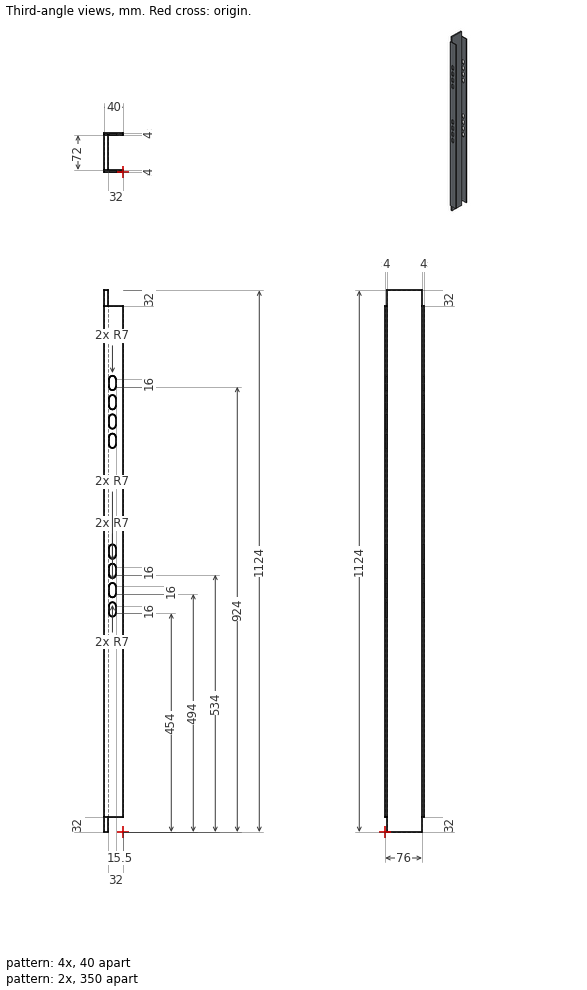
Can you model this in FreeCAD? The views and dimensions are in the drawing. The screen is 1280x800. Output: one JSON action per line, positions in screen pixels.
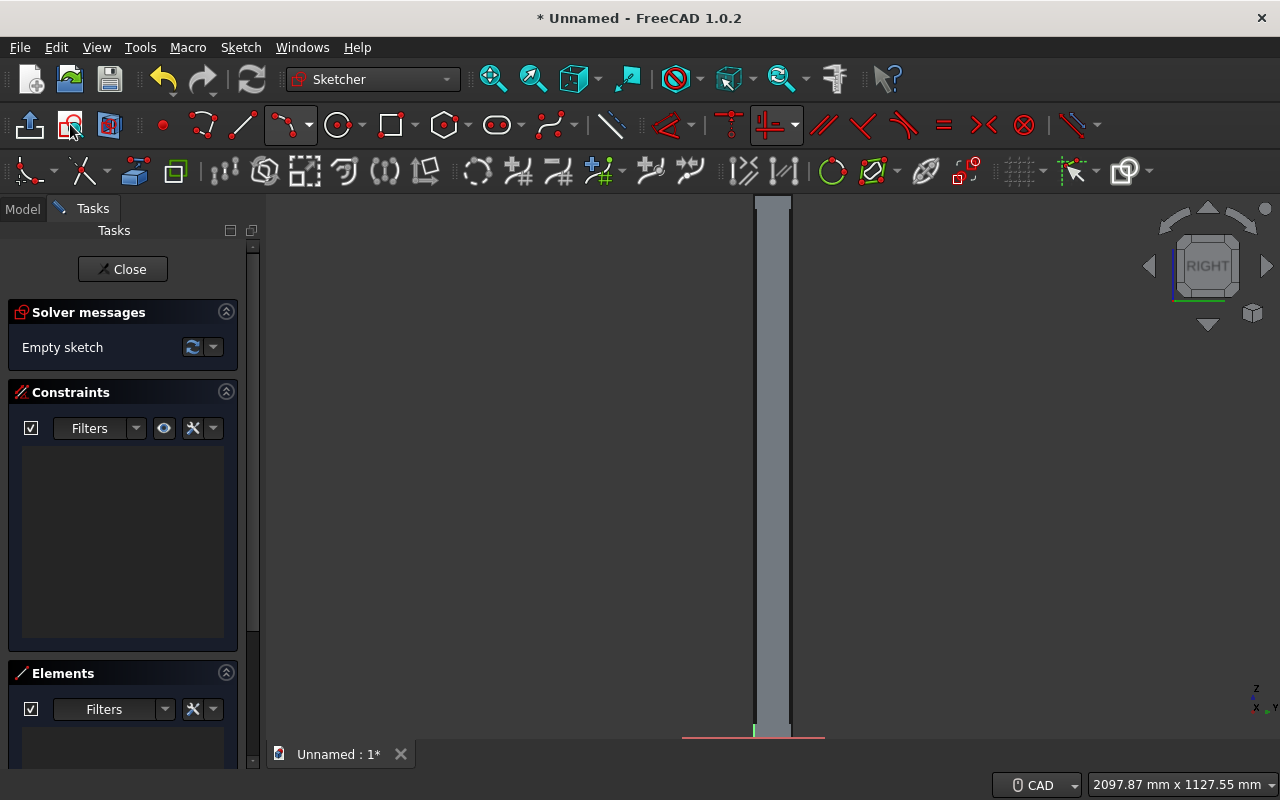
{"action": "scroll", "coordinate": [565, 466], "scroll_direction": "down", "scroll_amount": 2}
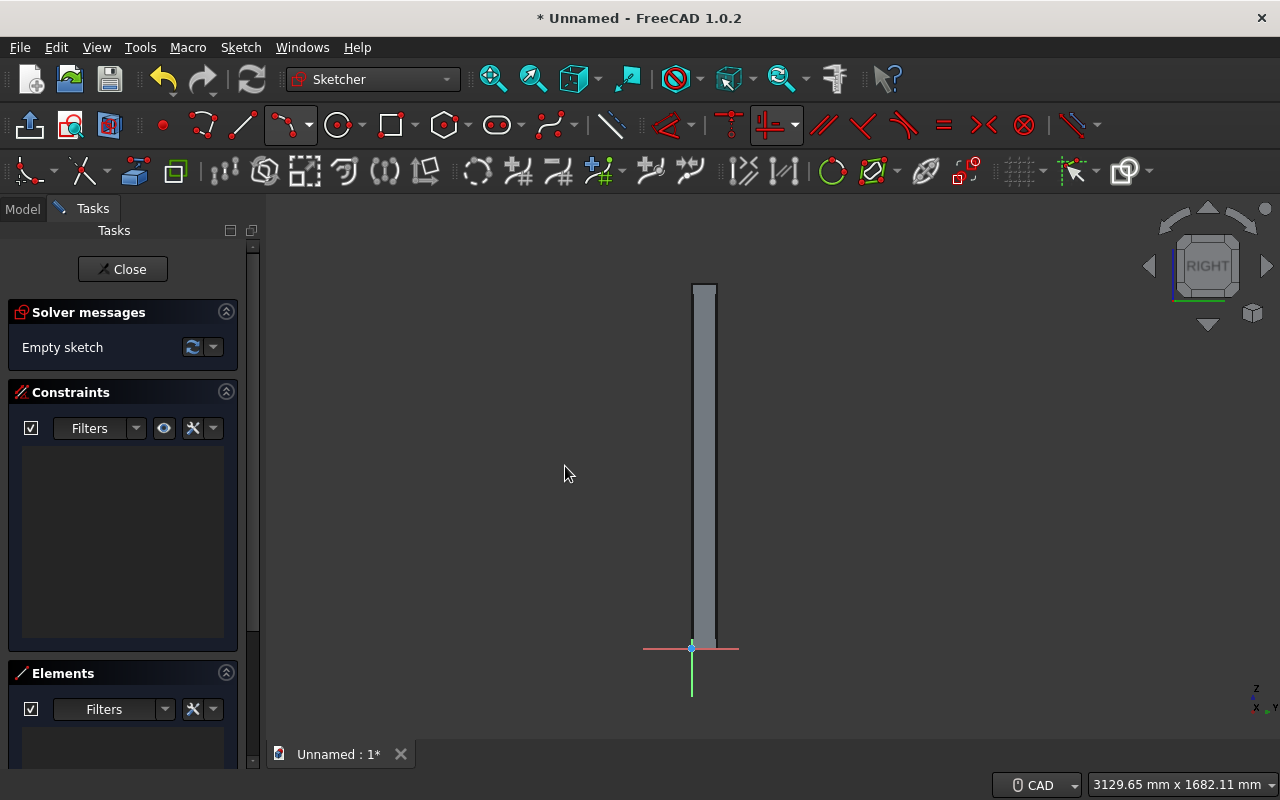
{"action": "key", "text": "g r"}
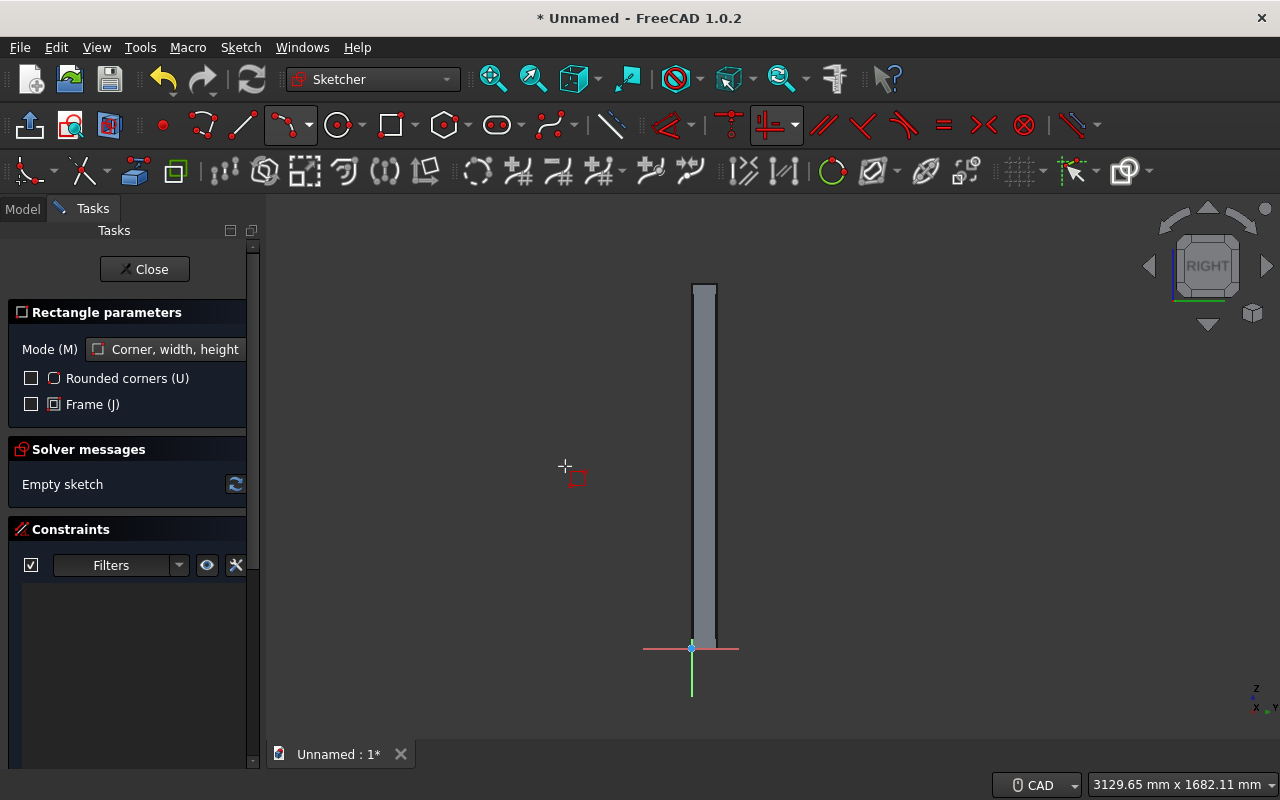
{"action": "scroll", "coordinate": [716, 284], "scroll_direction": "up", "scroll_amount": 13}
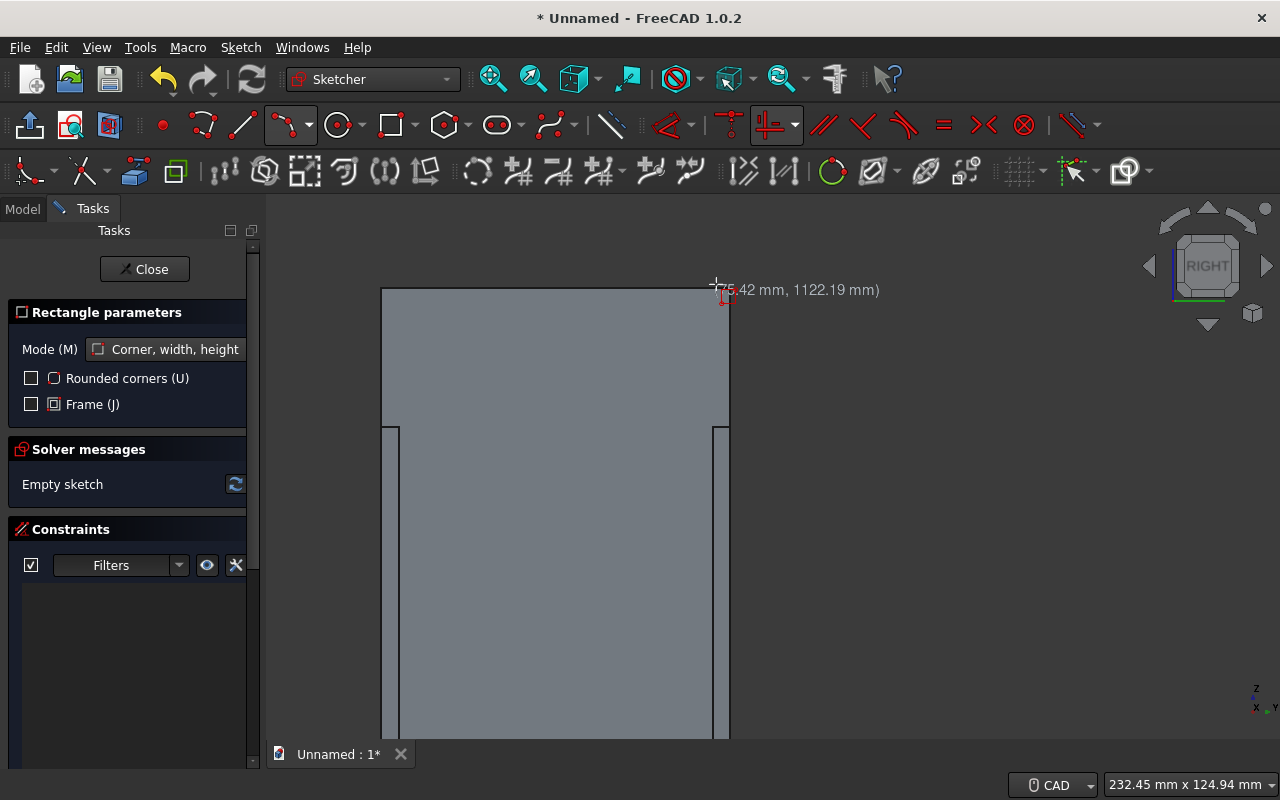
{"action": "scroll", "coordinate": [716, 284], "scroll_direction": "down", "scroll_amount": 13}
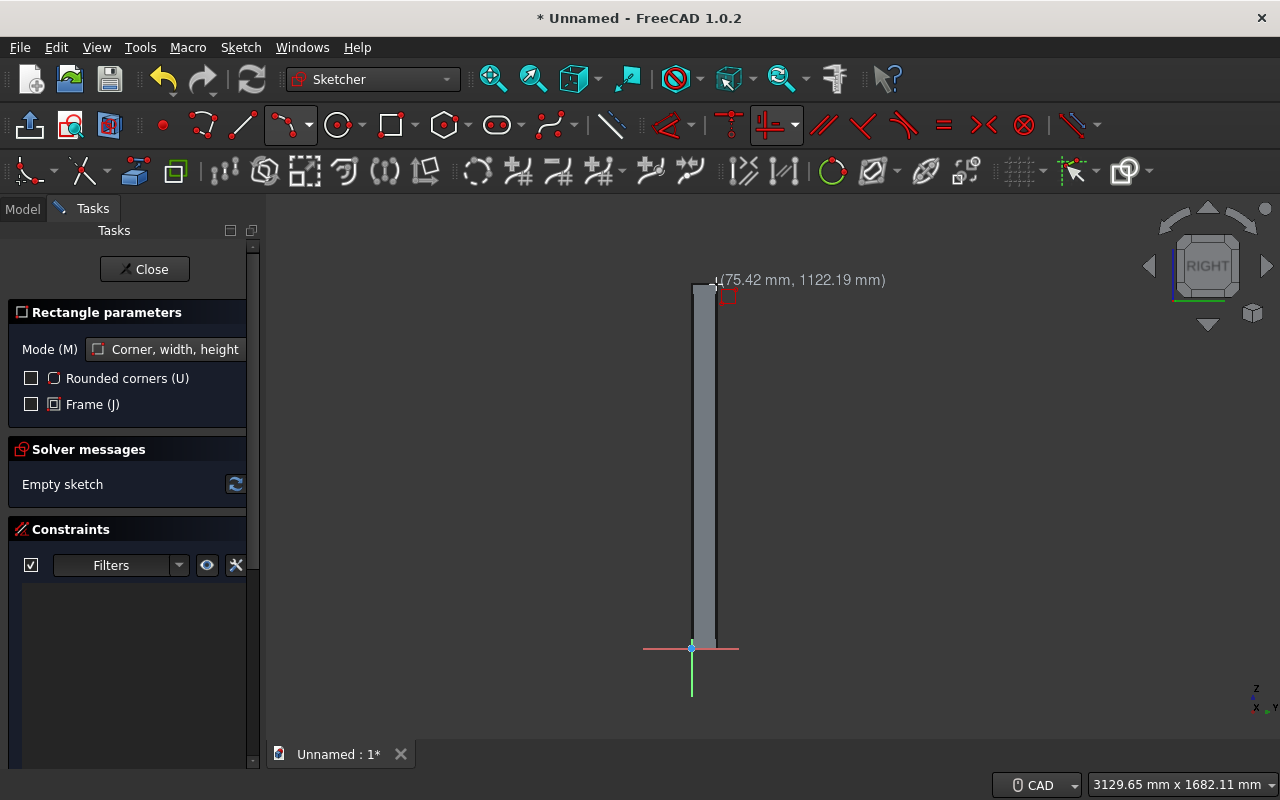
{"action": "left_click", "coordinate": [716, 284]}
{"action": "left_click", "coordinate": [717, 295]}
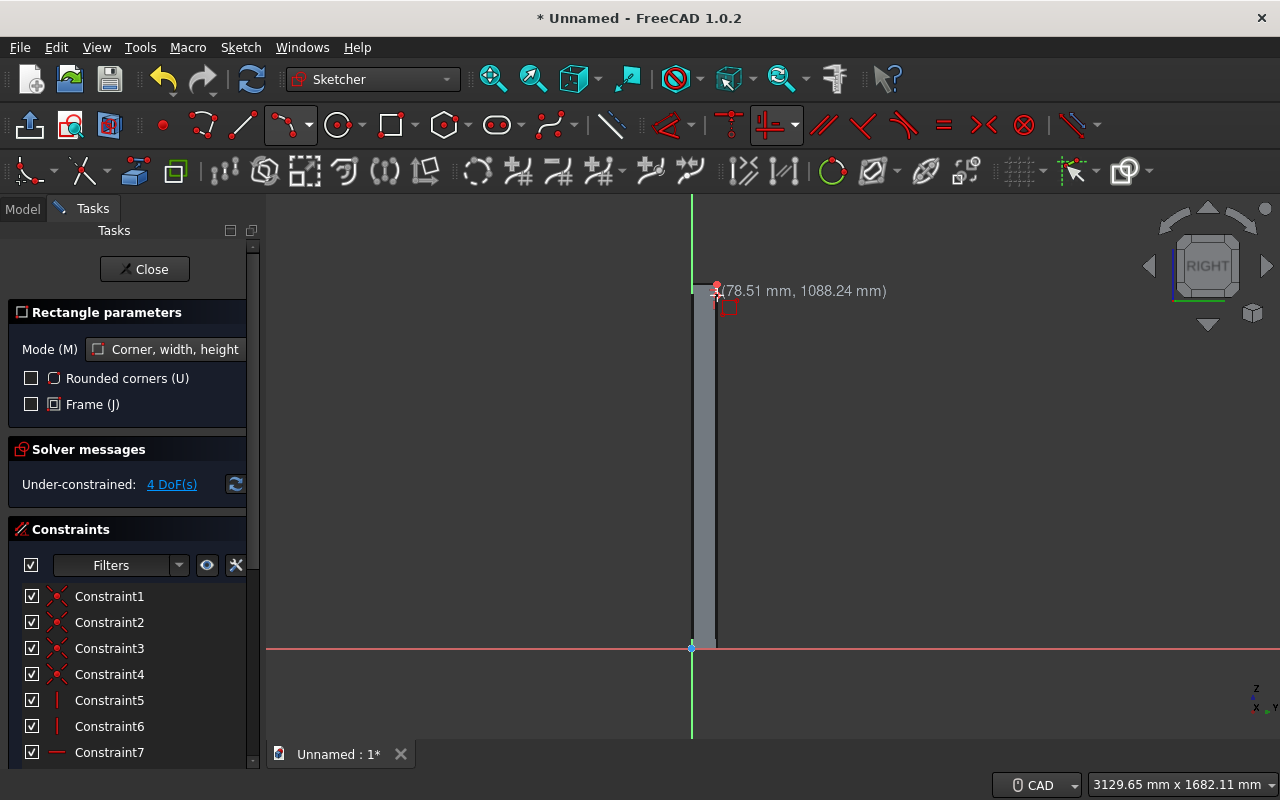
{"action": "scroll", "coordinate": [692, 284], "scroll_direction": "up", "scroll_amount": 13}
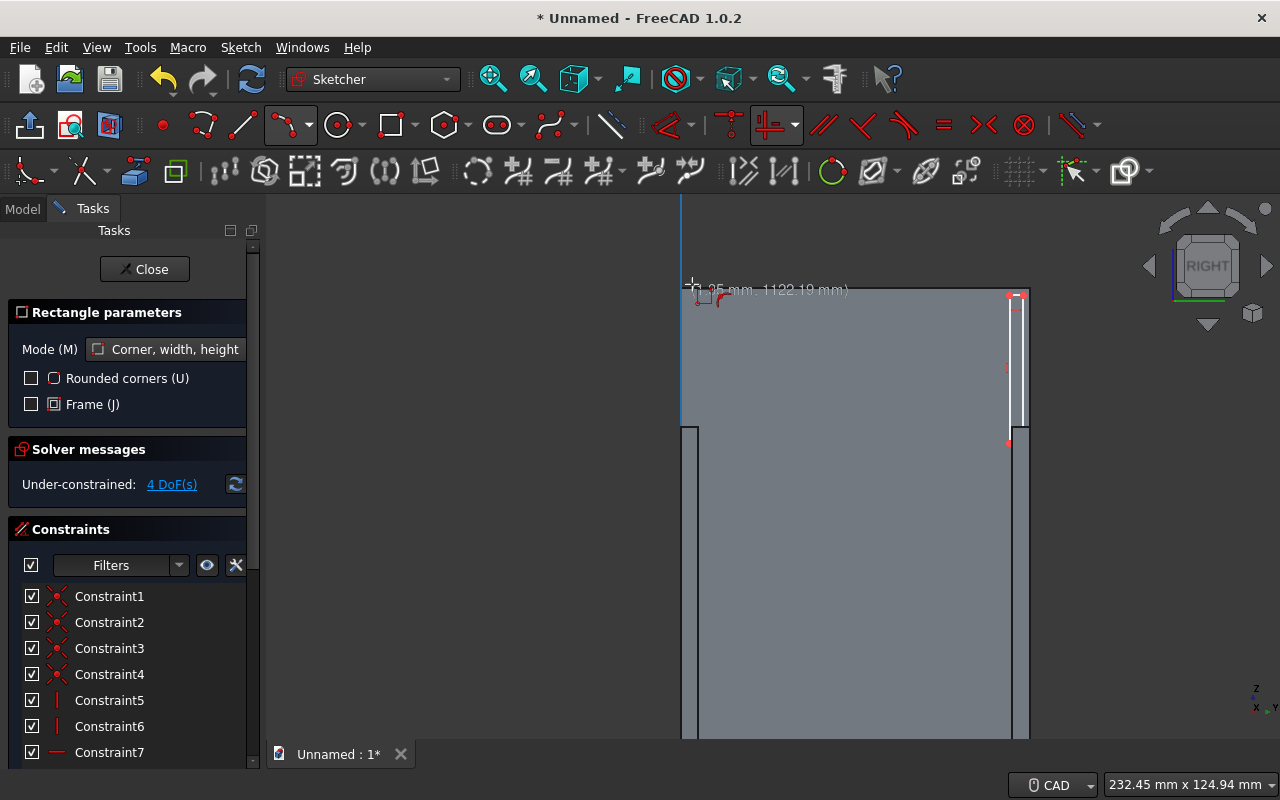
{"action": "scroll", "coordinate": [692, 284], "scroll_direction": "down", "scroll_amount": 13}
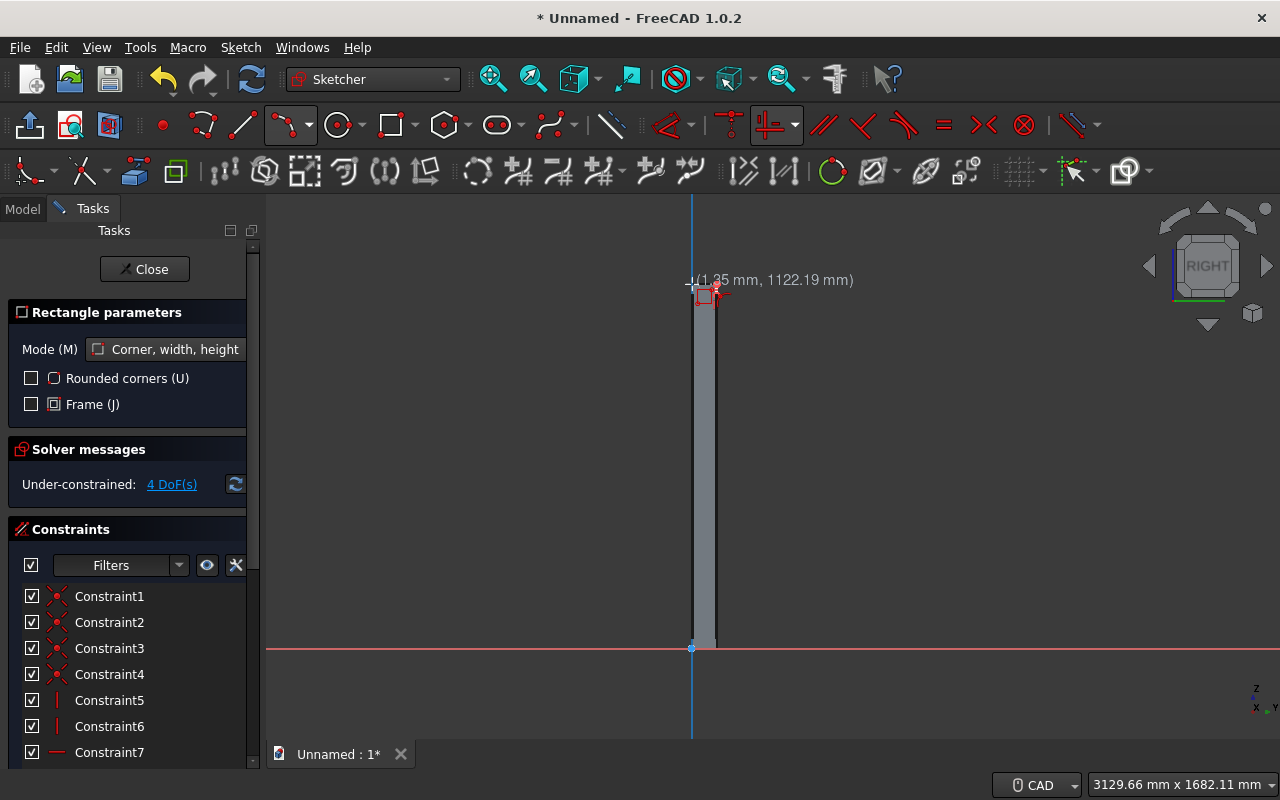
{"action": "left_click", "coordinate": [692, 284]}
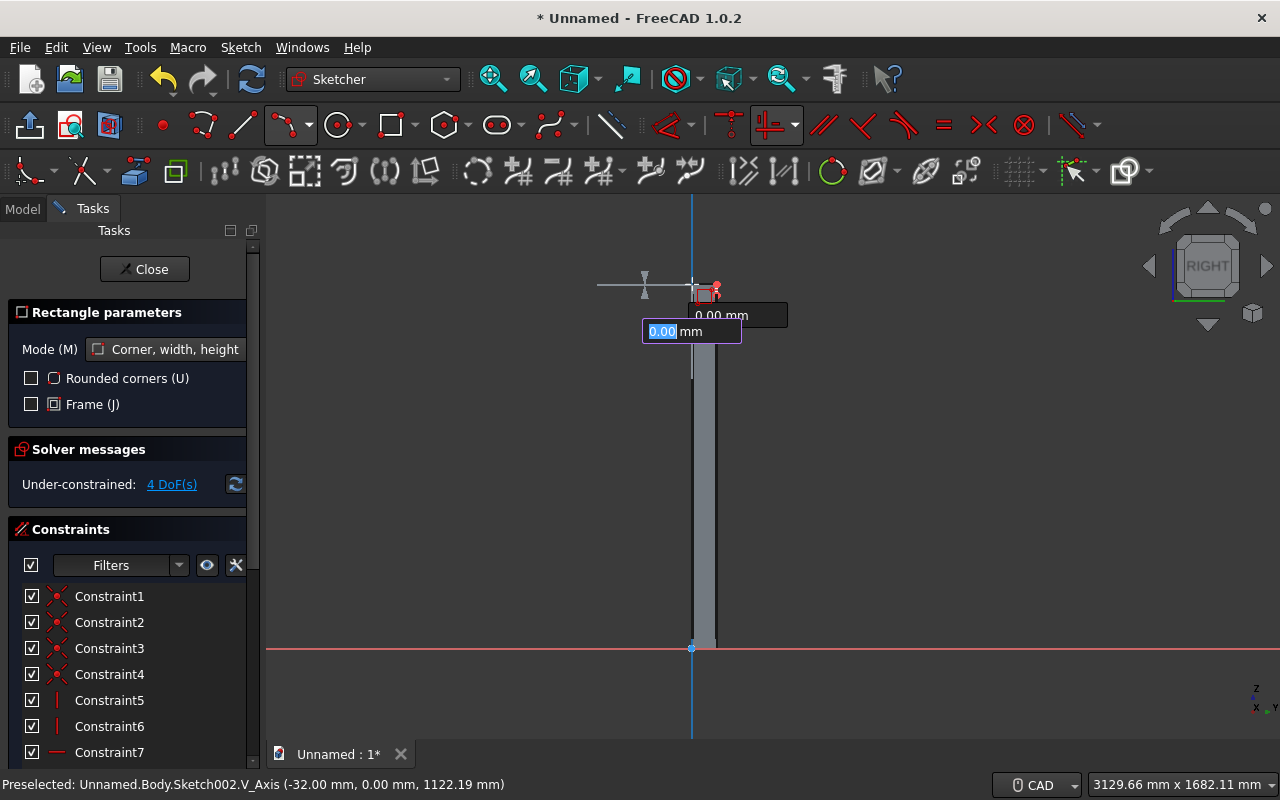
{"action": "scroll", "coordinate": [693, 295], "scroll_direction": "up", "scroll_amount": 13}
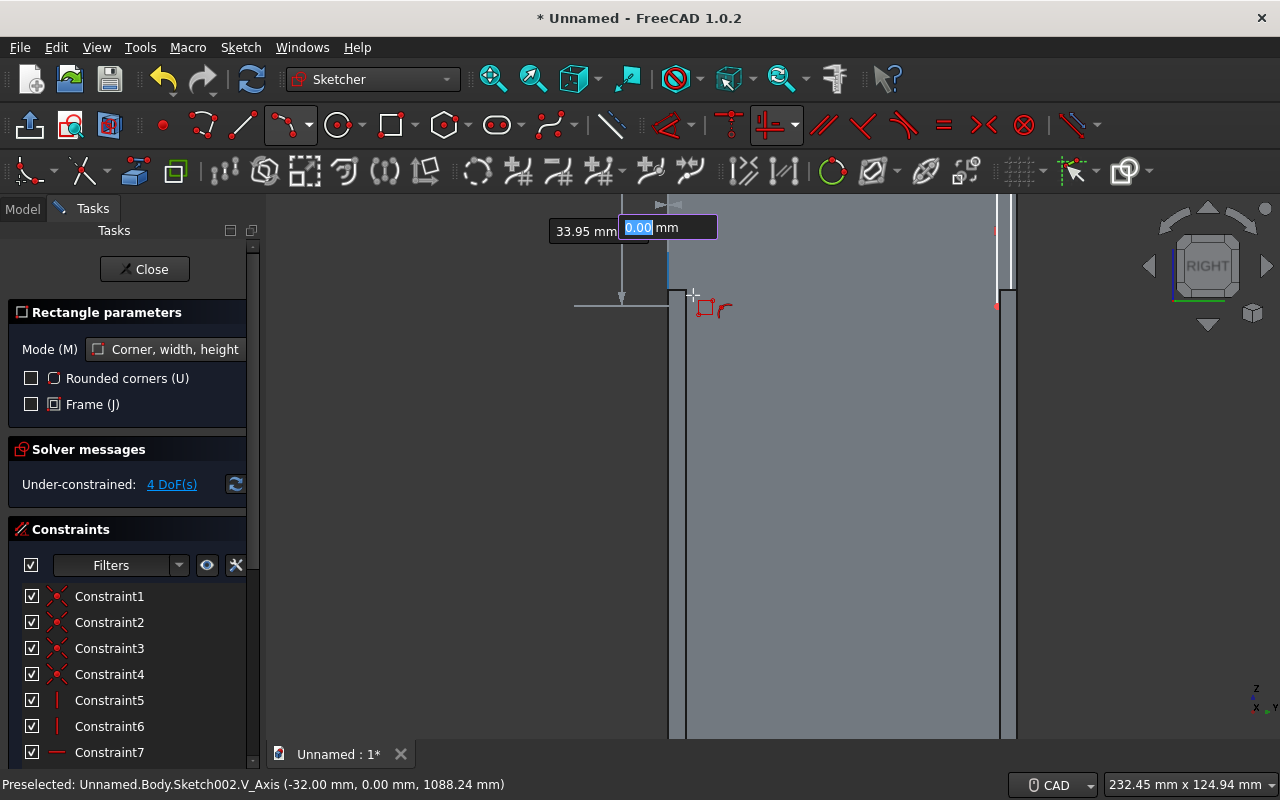
{"action": "left_click", "coordinate": [686, 290]}